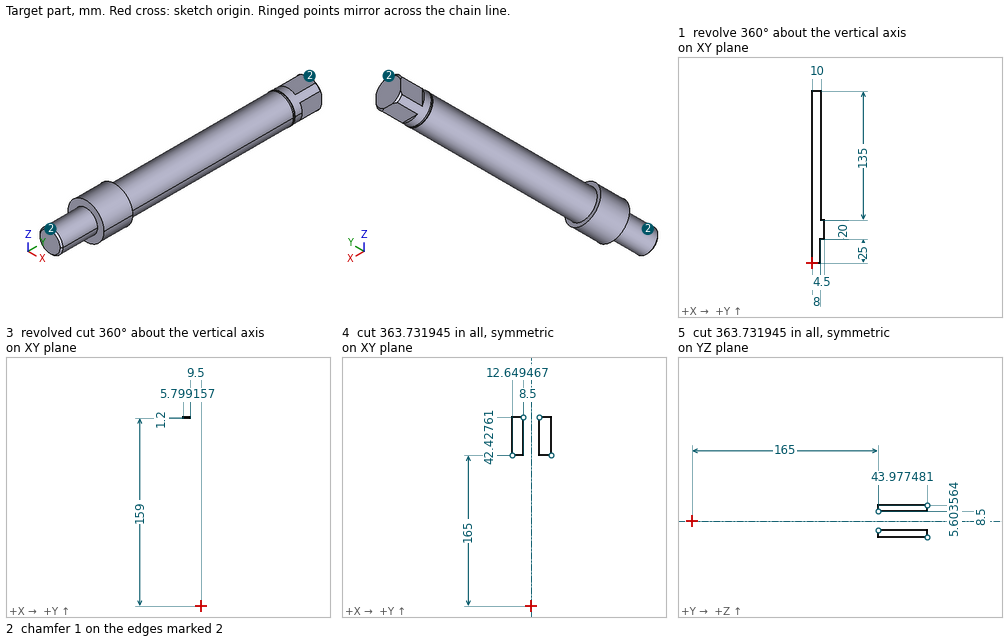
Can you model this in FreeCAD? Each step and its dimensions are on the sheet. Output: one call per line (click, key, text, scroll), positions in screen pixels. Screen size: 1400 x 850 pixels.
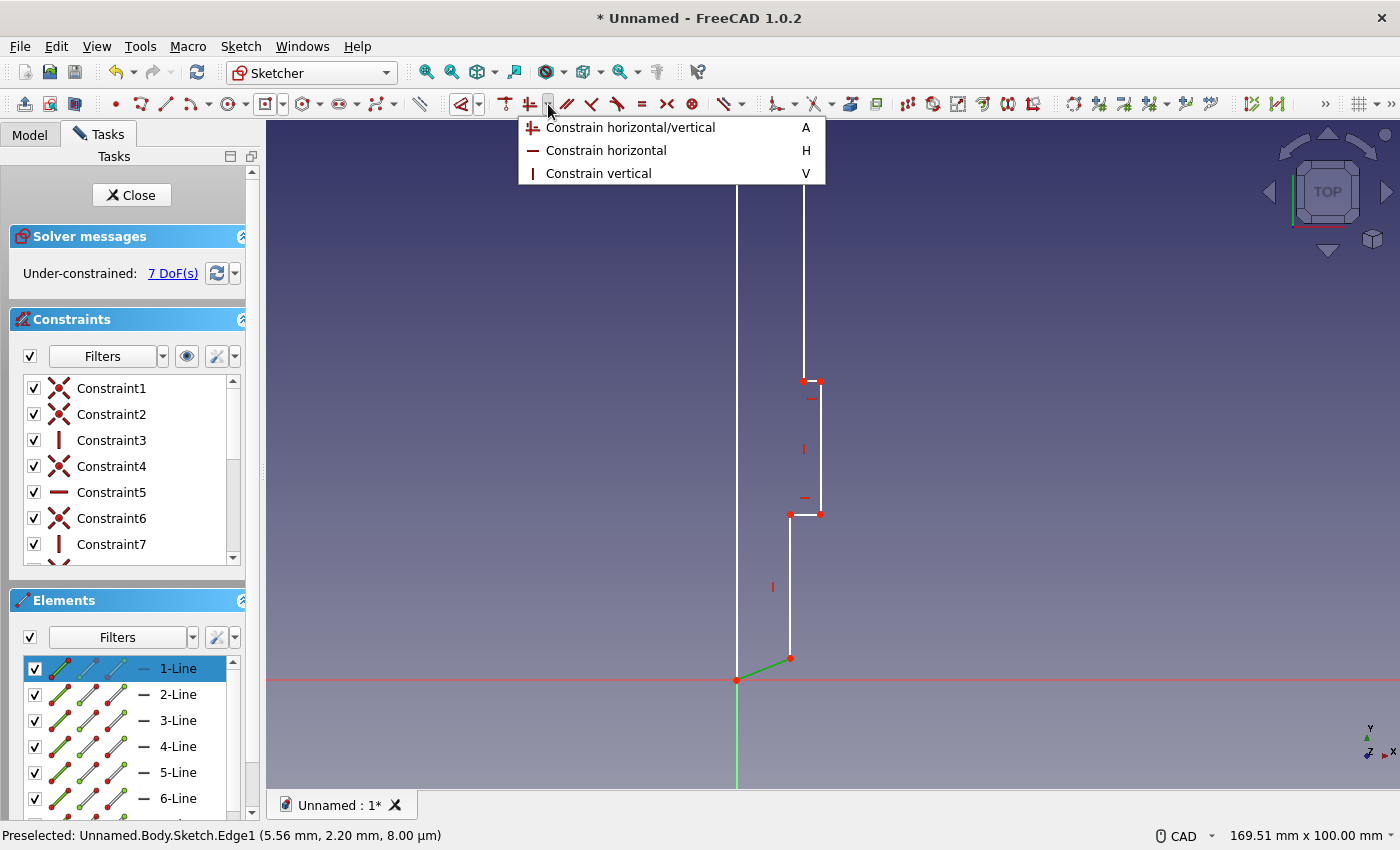
click(672, 150)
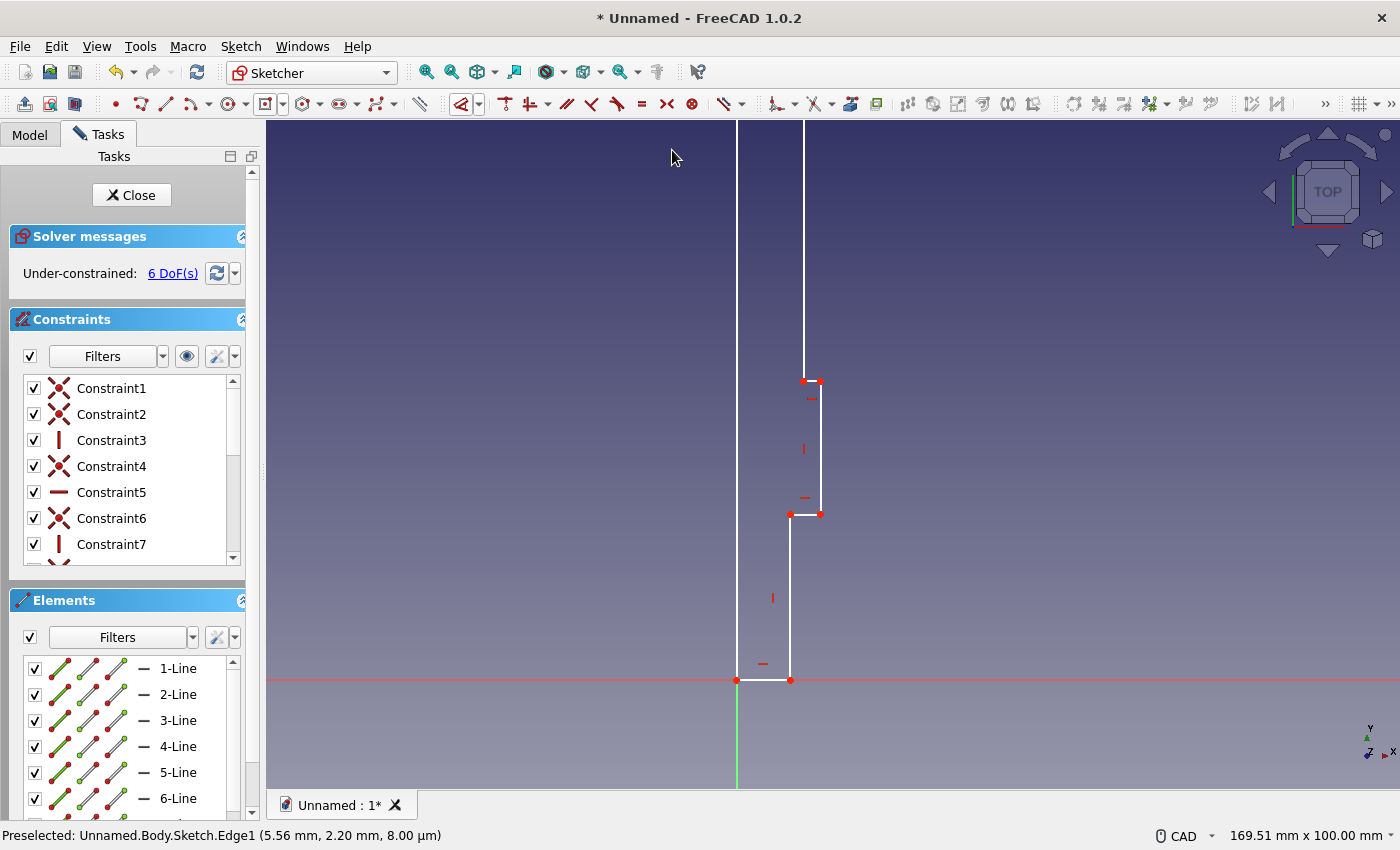
key(d)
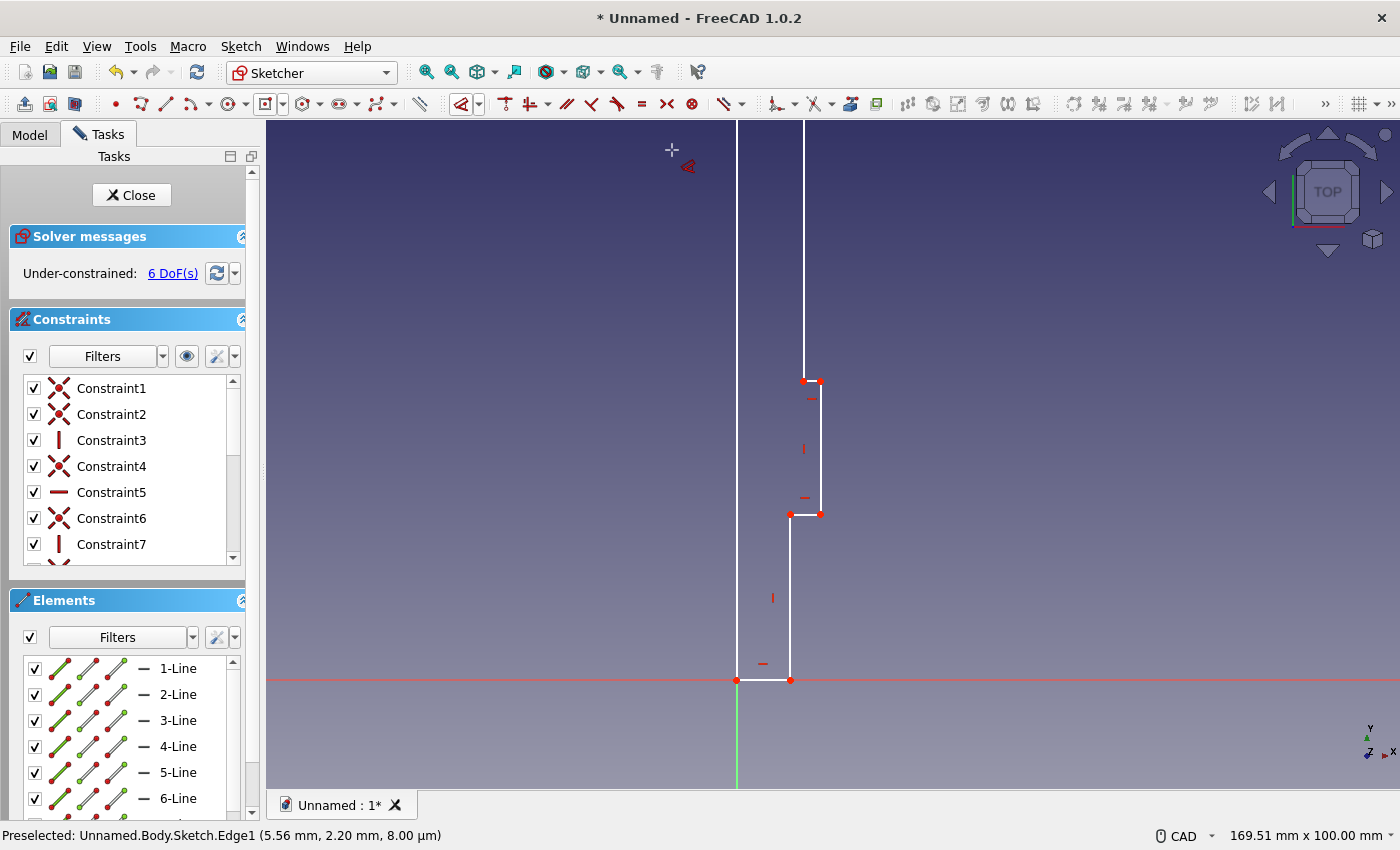
click(753, 680)
click(763, 714)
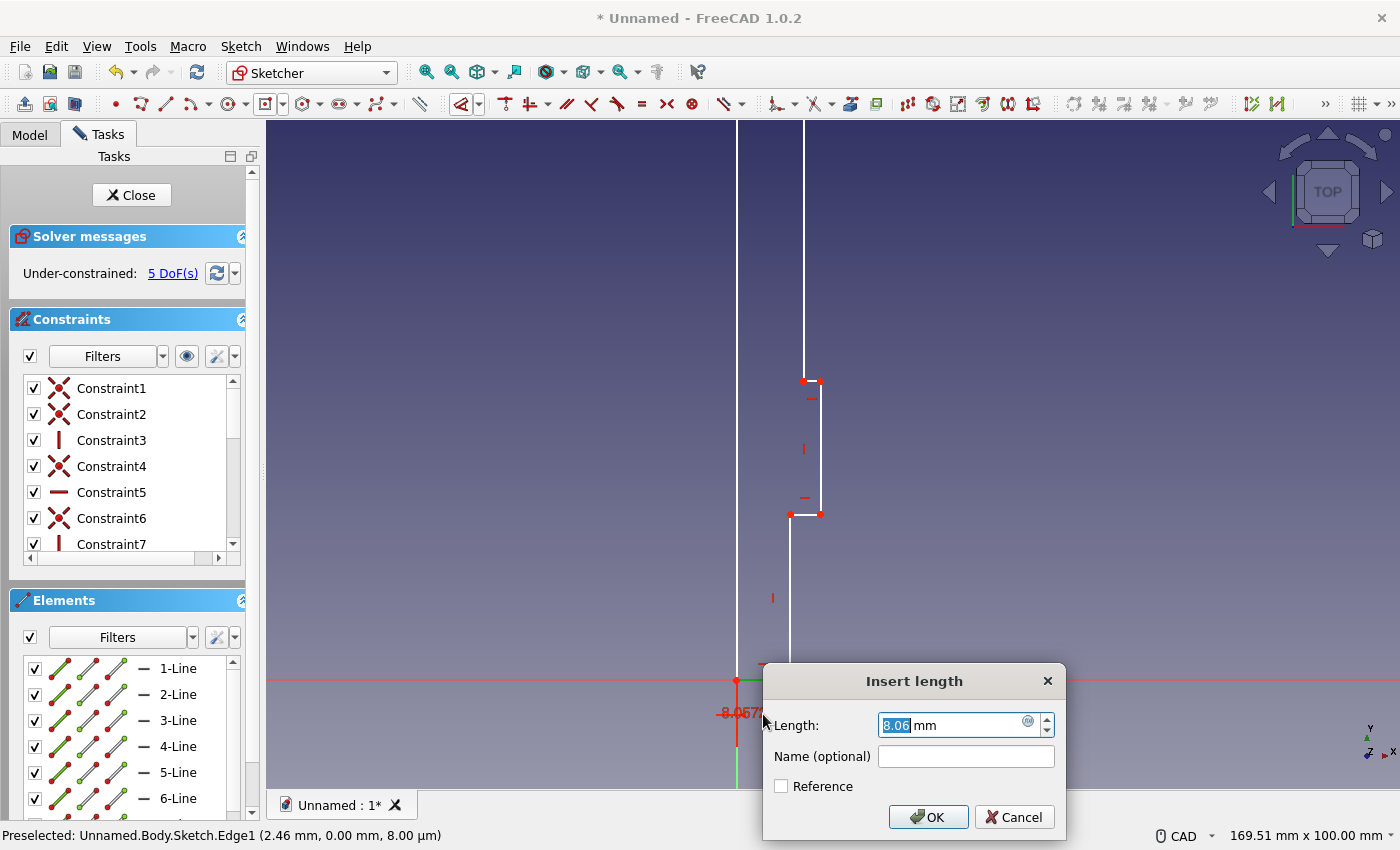
text(8)
key(Return)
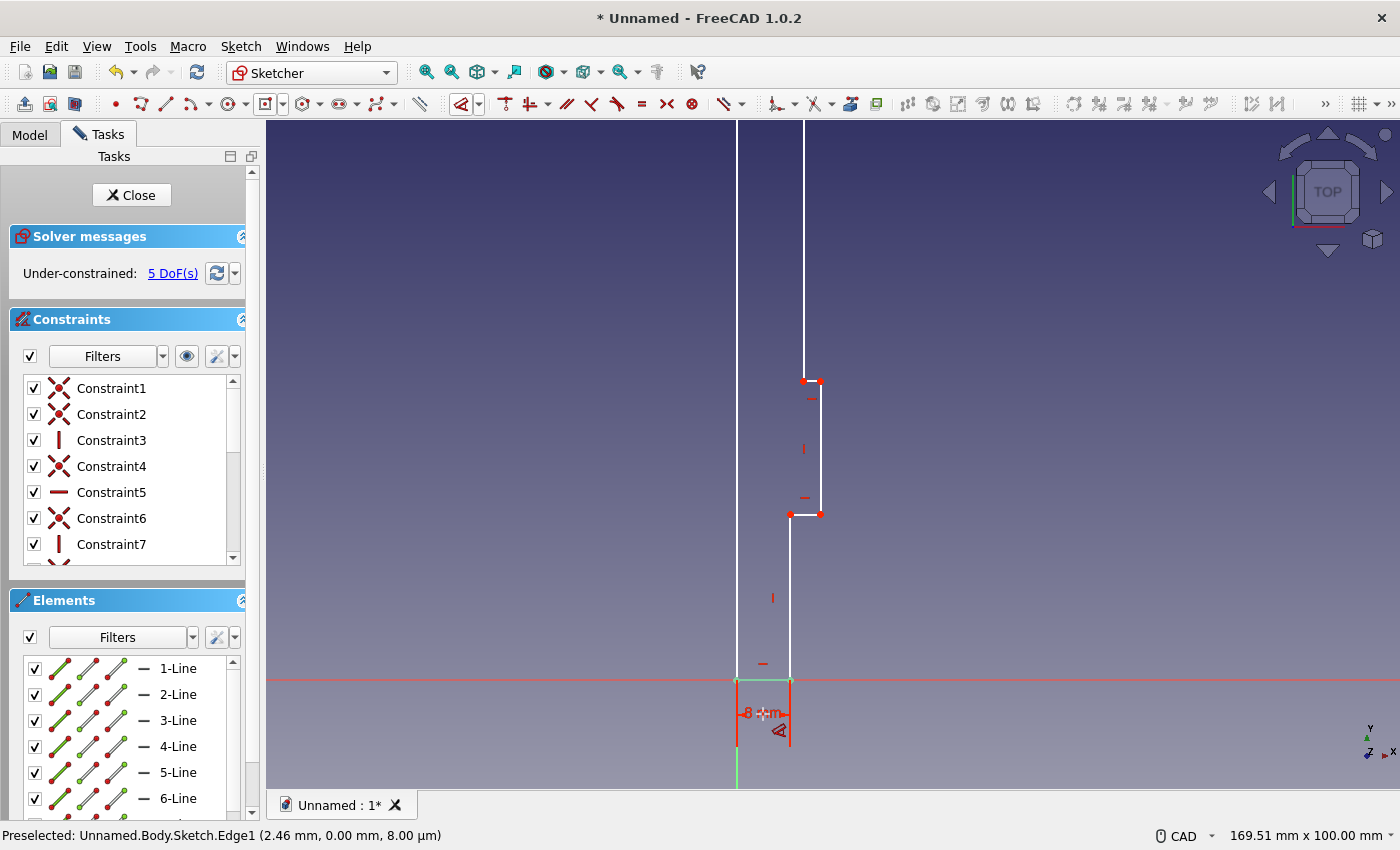
click(790, 630)
click(824, 597)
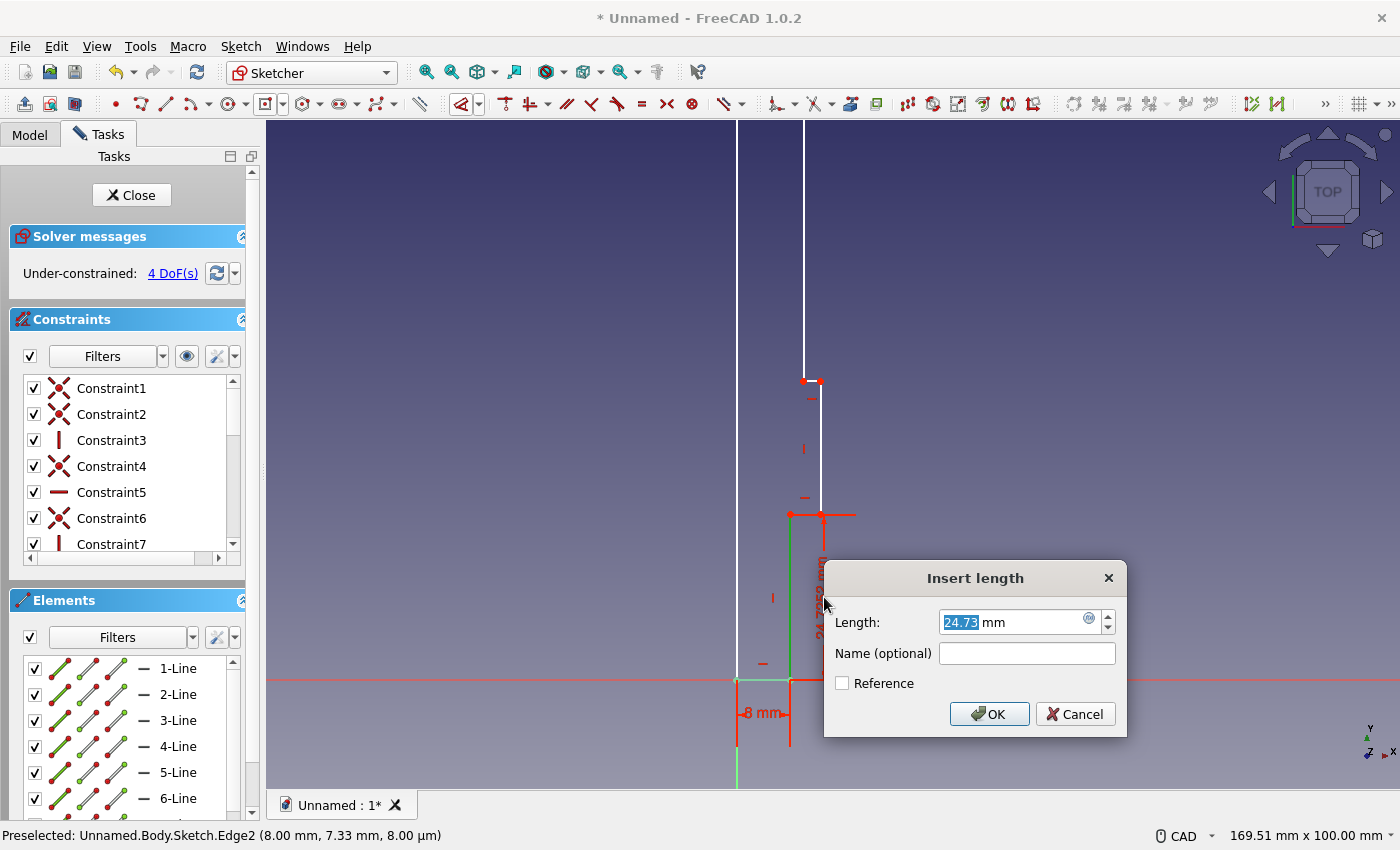
text(25)
key(Return)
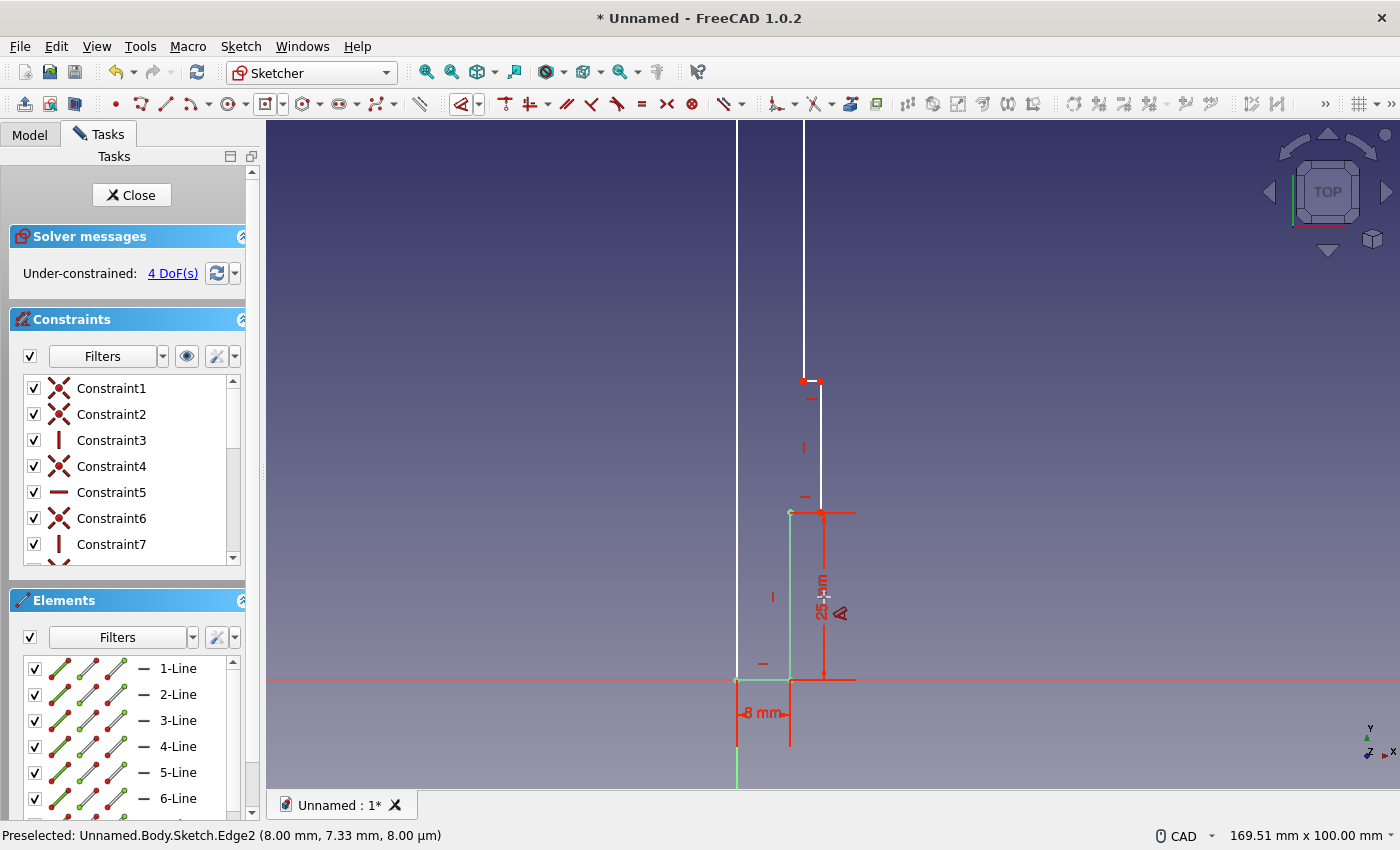
click(821, 473)
click(855, 447)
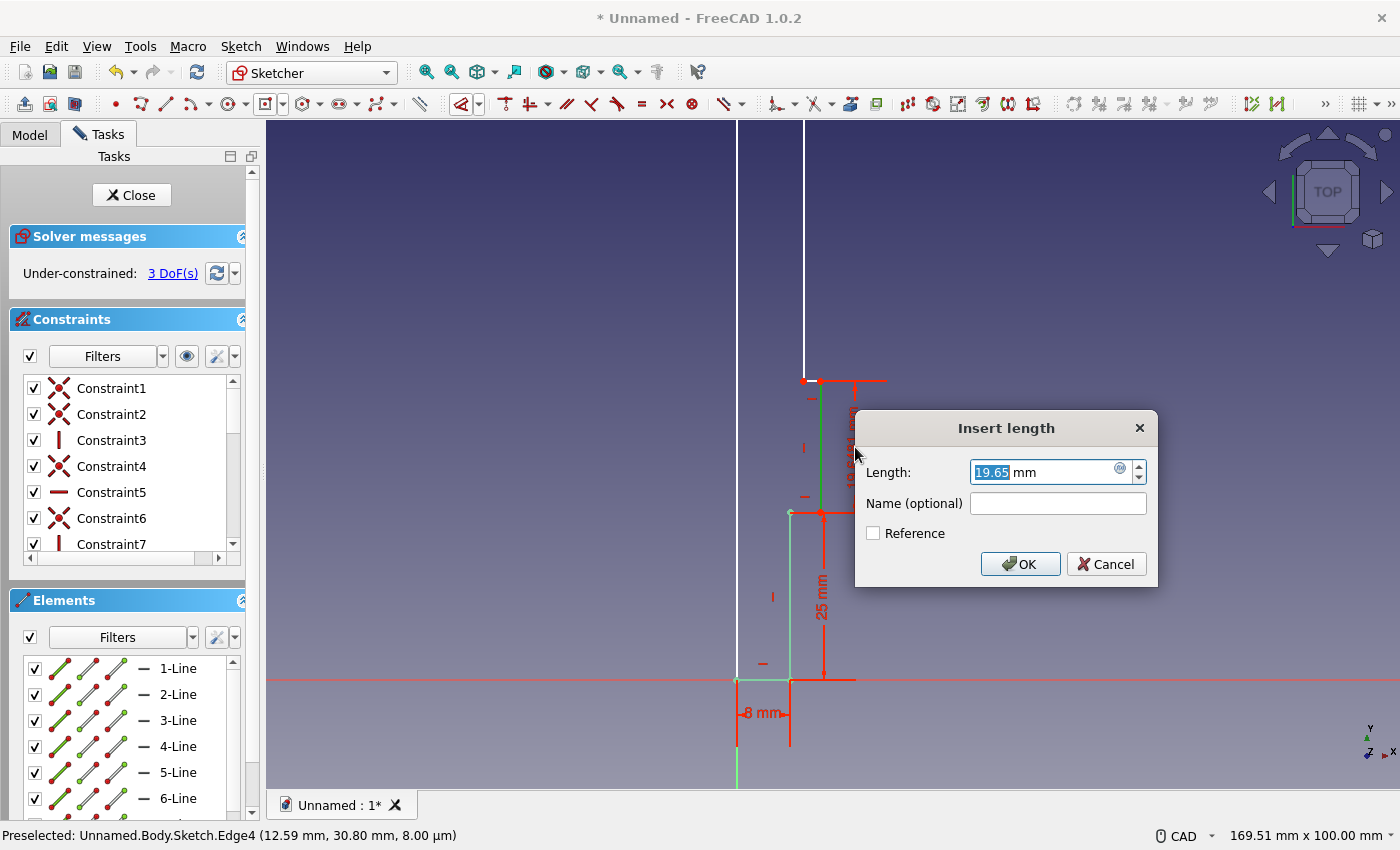
text(20)
key(Return)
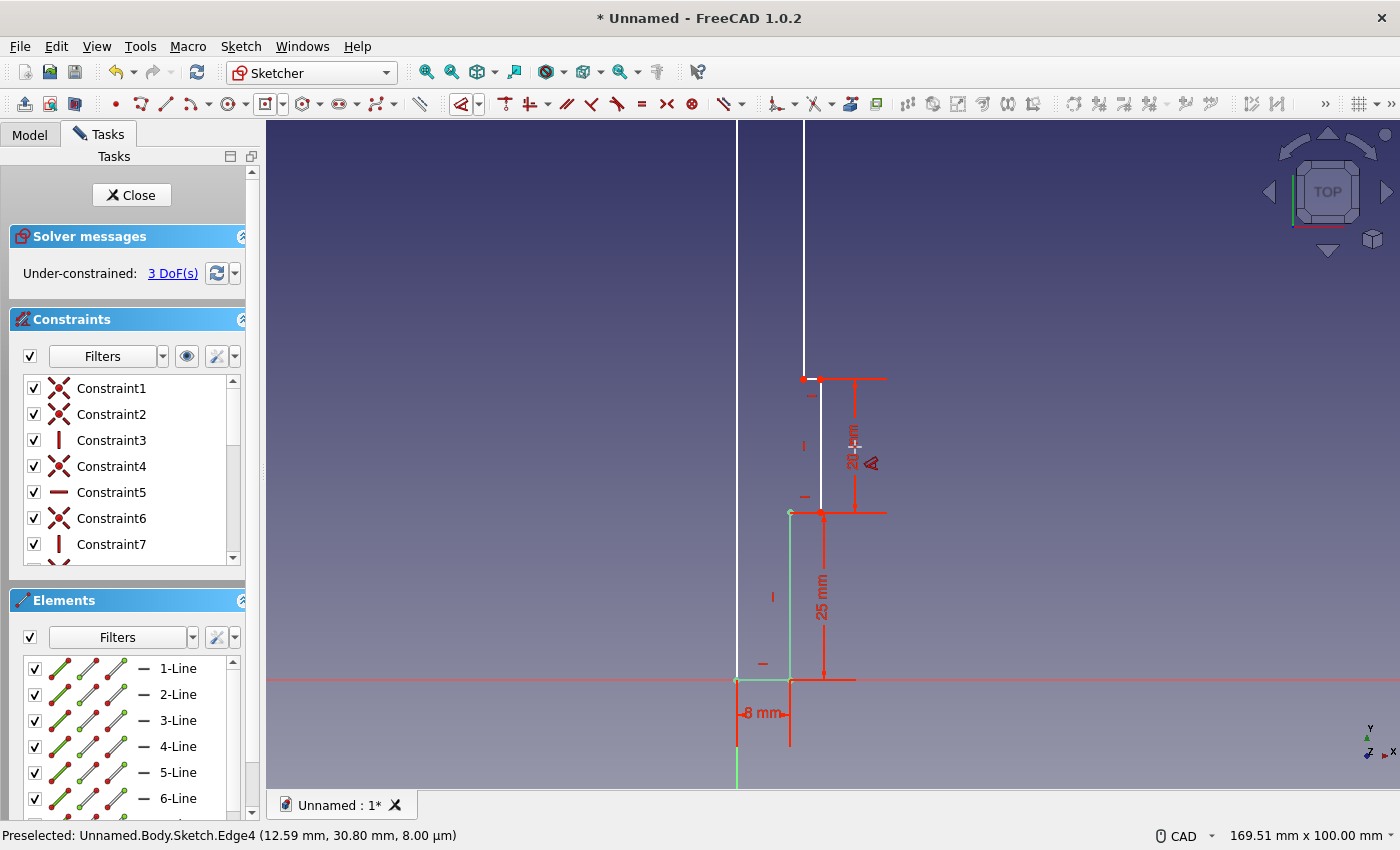
scroll(756, 674, down, 5)